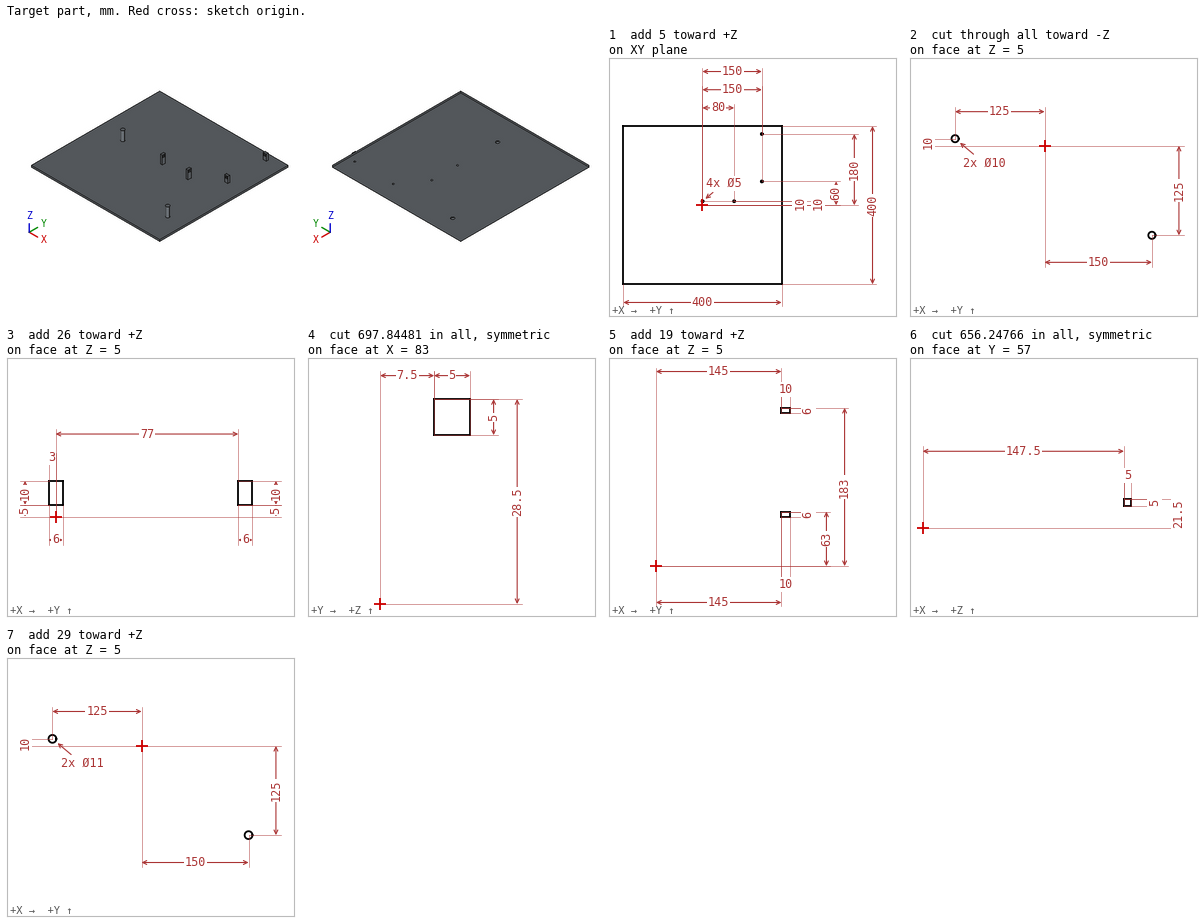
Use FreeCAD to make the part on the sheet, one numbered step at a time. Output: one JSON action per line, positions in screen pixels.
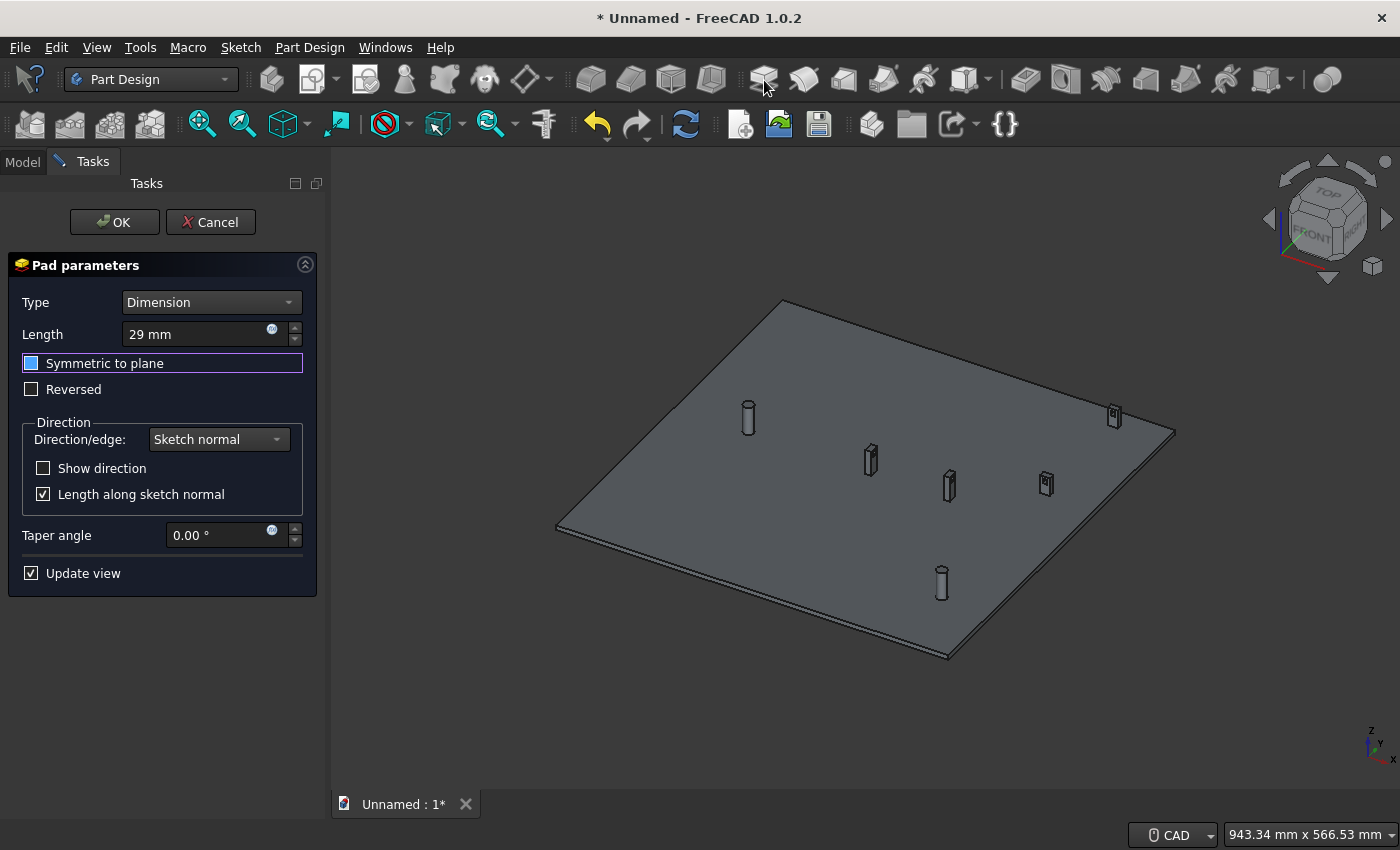
{"action": "left_click", "coordinate": [115, 222]}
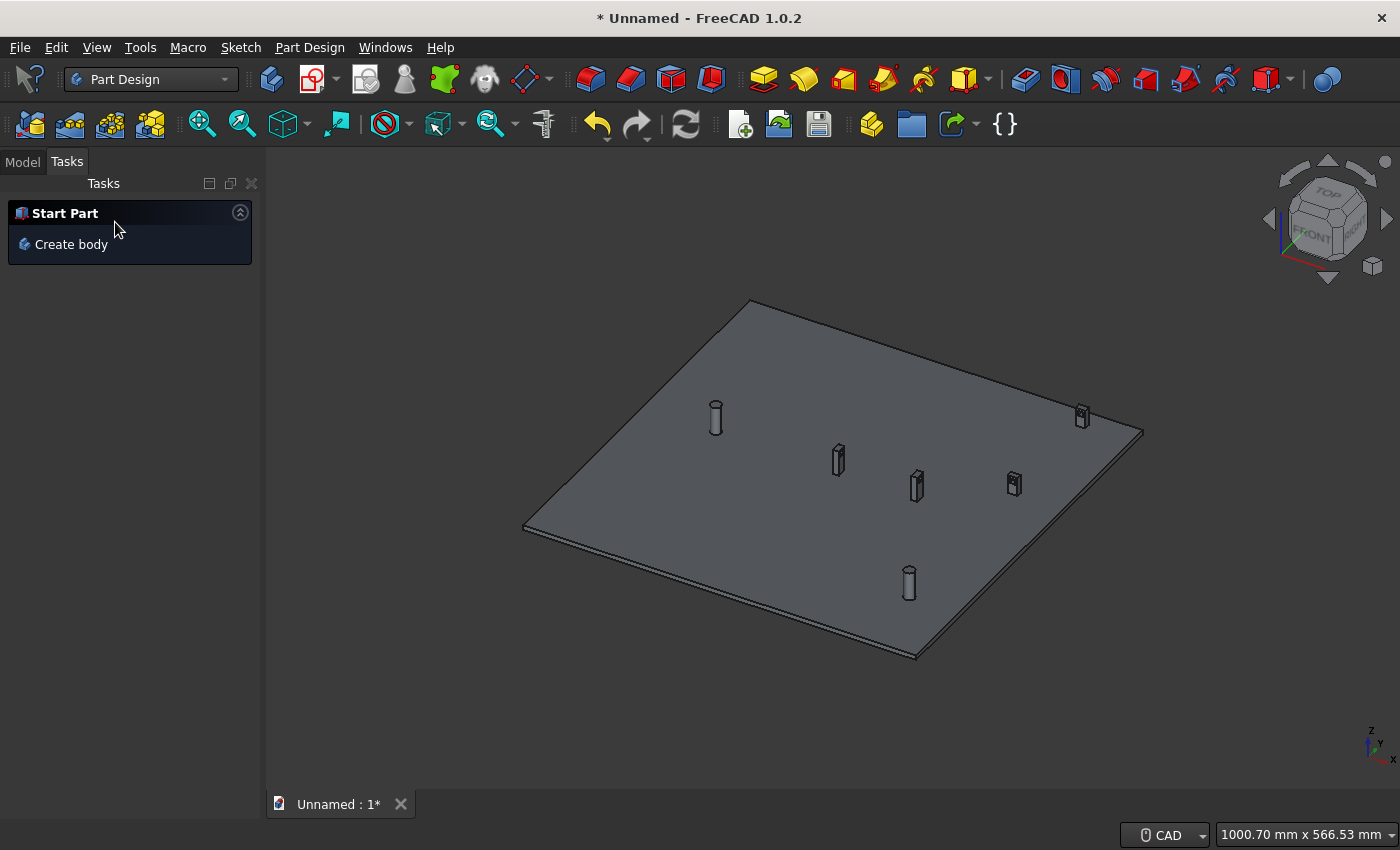
{"action": "key", "text": "0"}